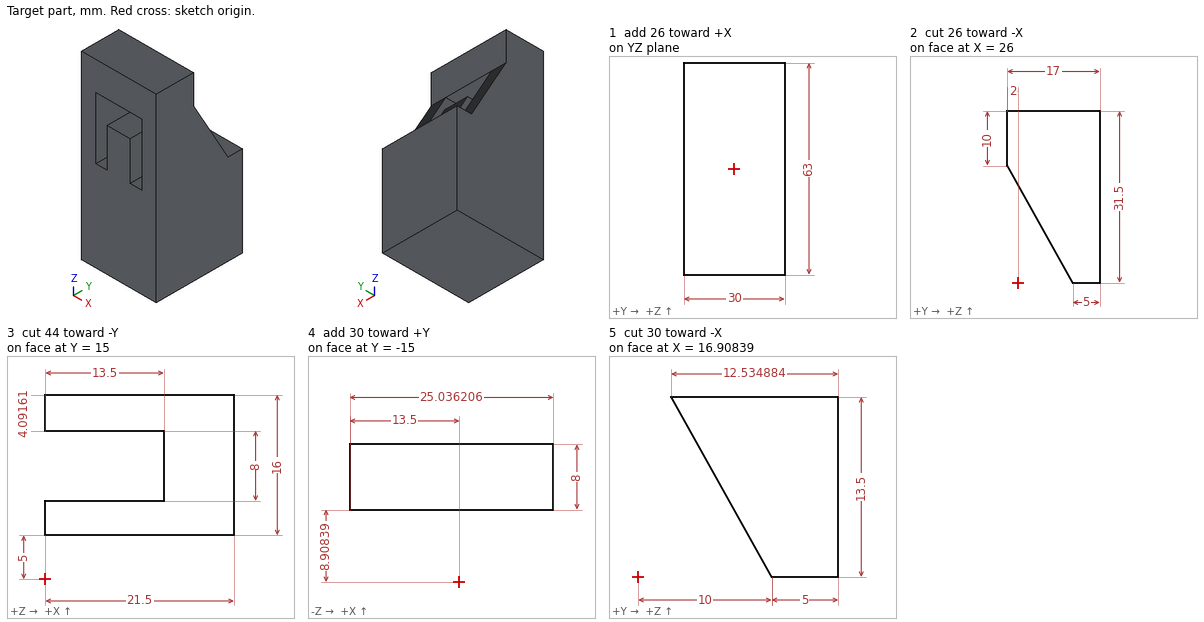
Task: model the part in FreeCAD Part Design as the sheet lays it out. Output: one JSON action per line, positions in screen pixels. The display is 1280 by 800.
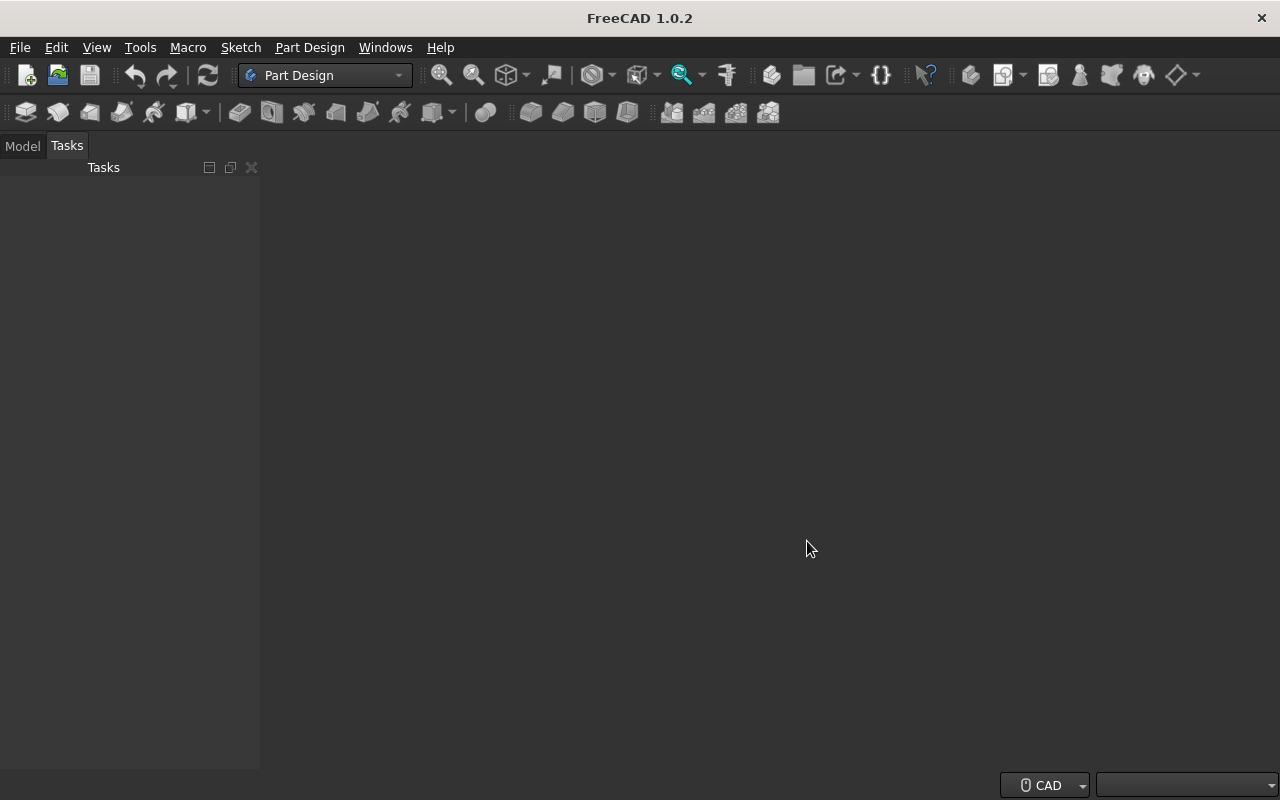
{"action": "key", "text": "ctrl+n"}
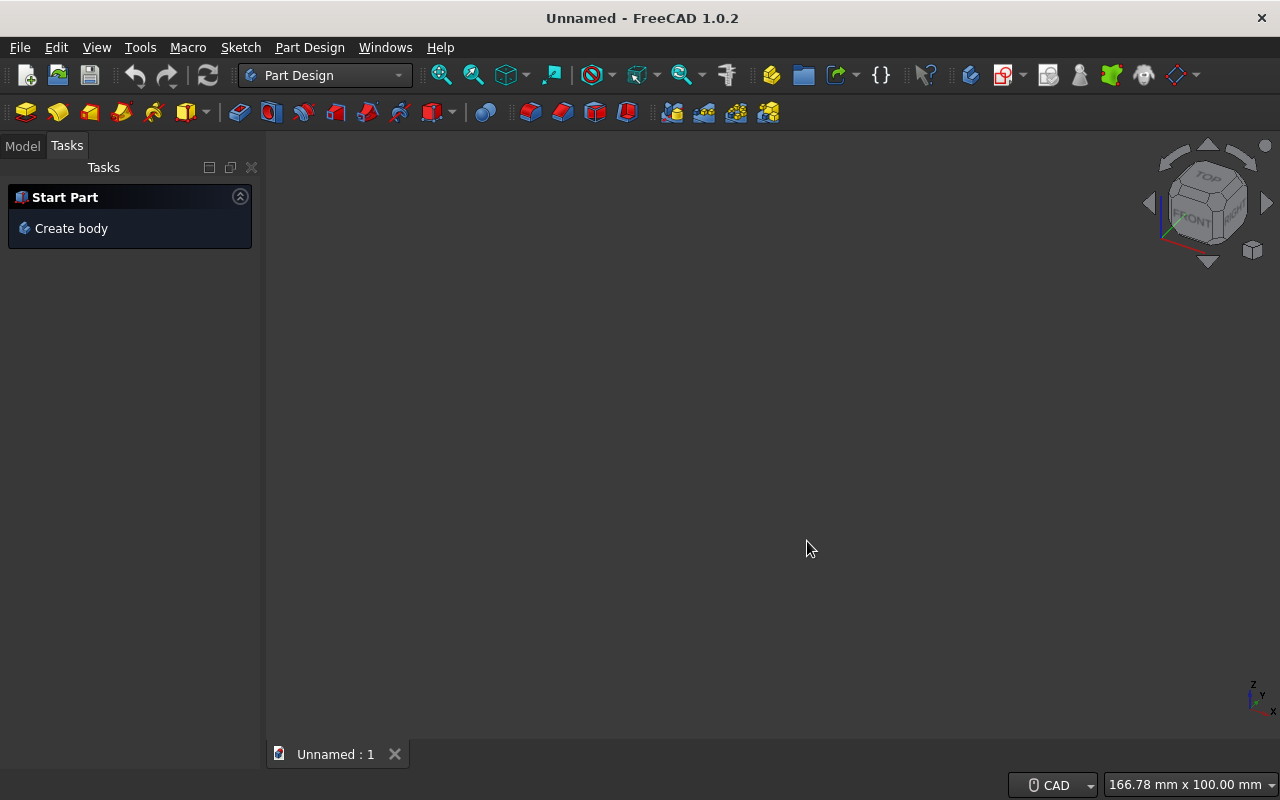
{"action": "left_click", "coordinate": [1004, 76]}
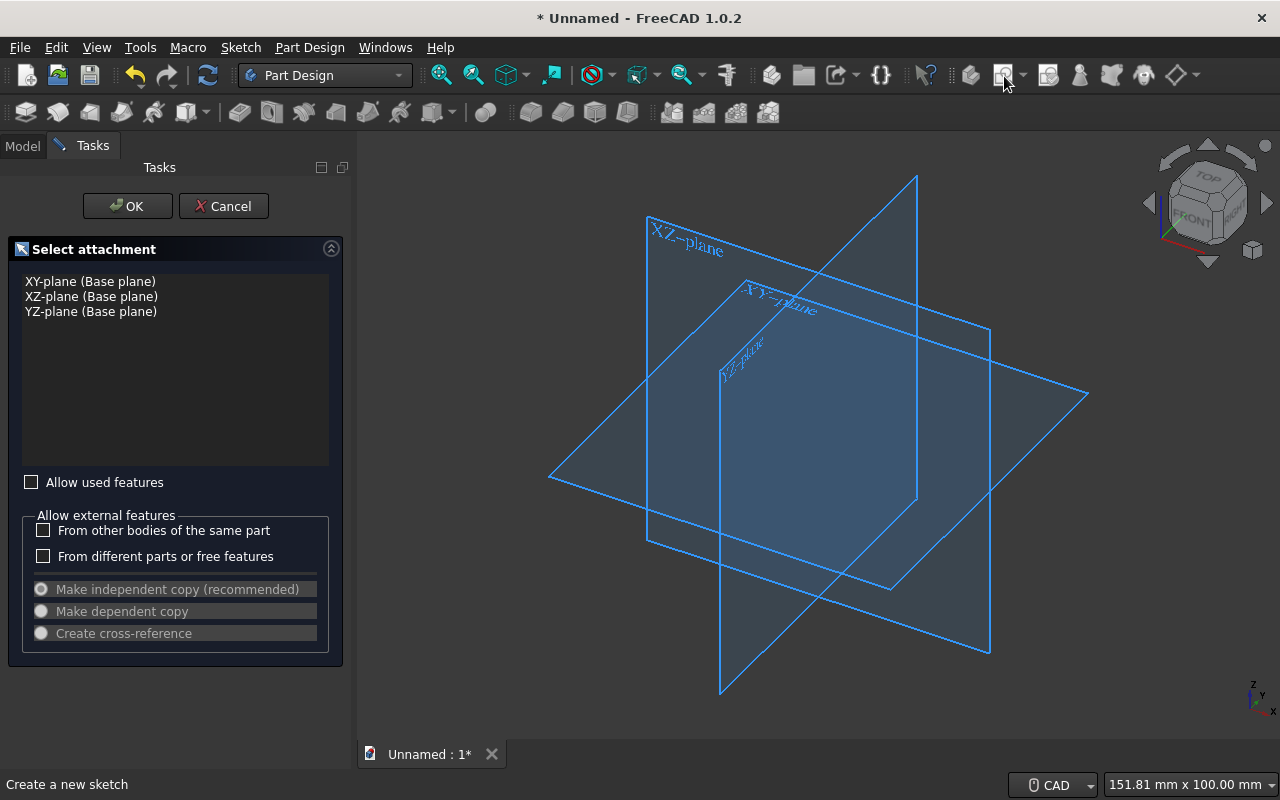
{"action": "left_click", "coordinate": [82, 312]}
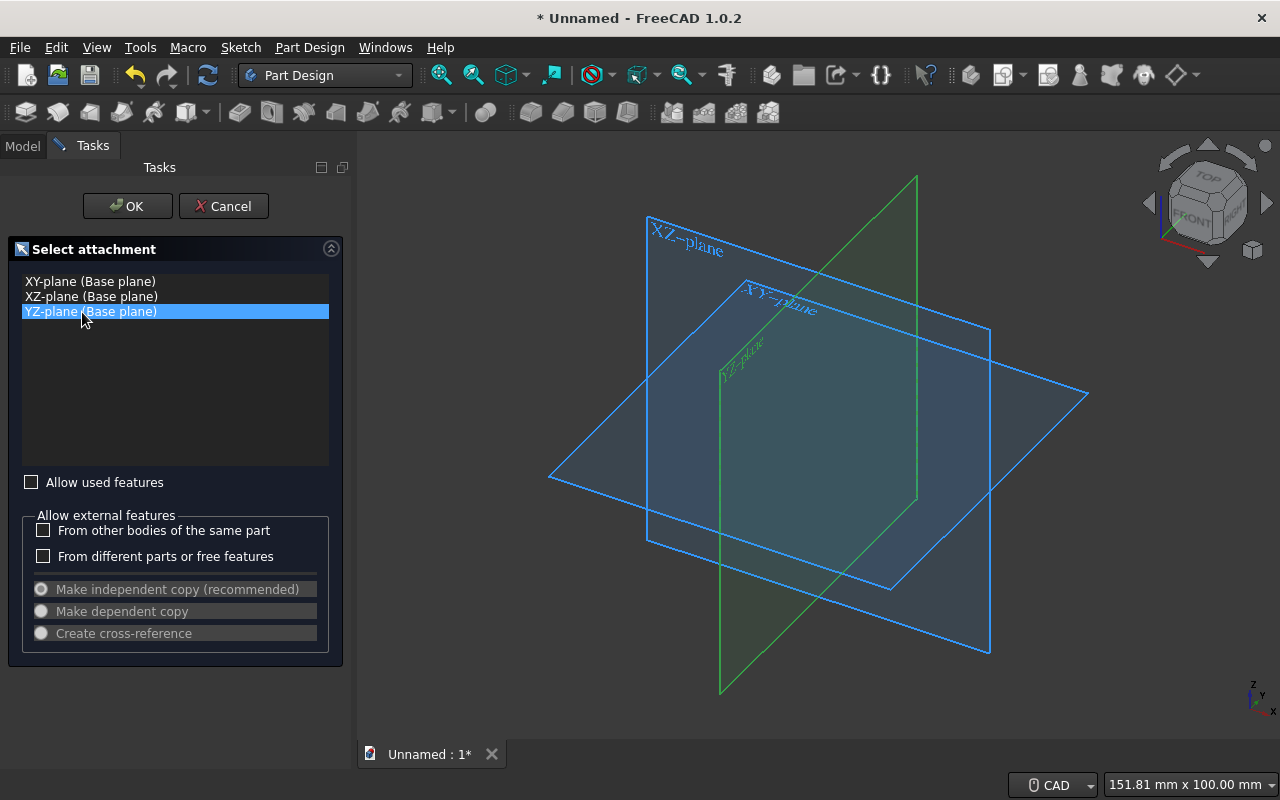
{"action": "left_click", "coordinate": [128, 206]}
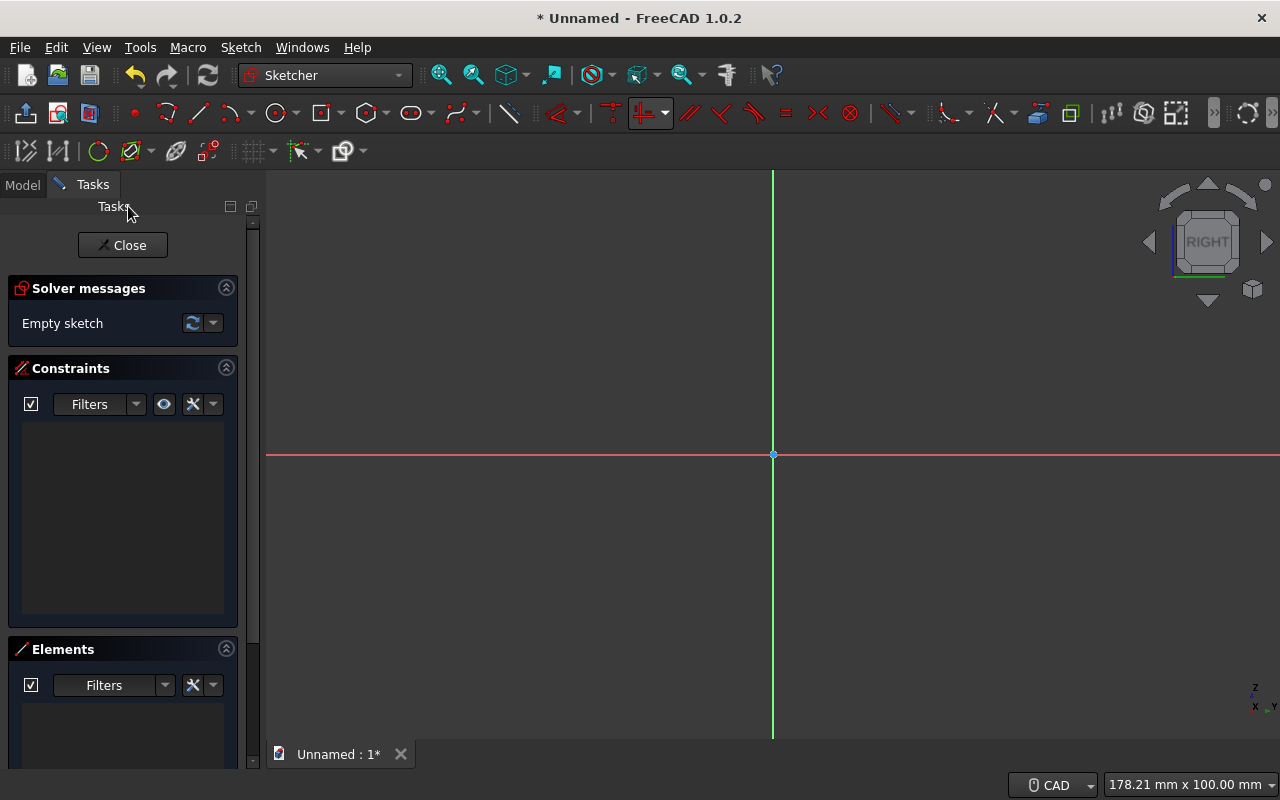
{"action": "key", "text": "g v"}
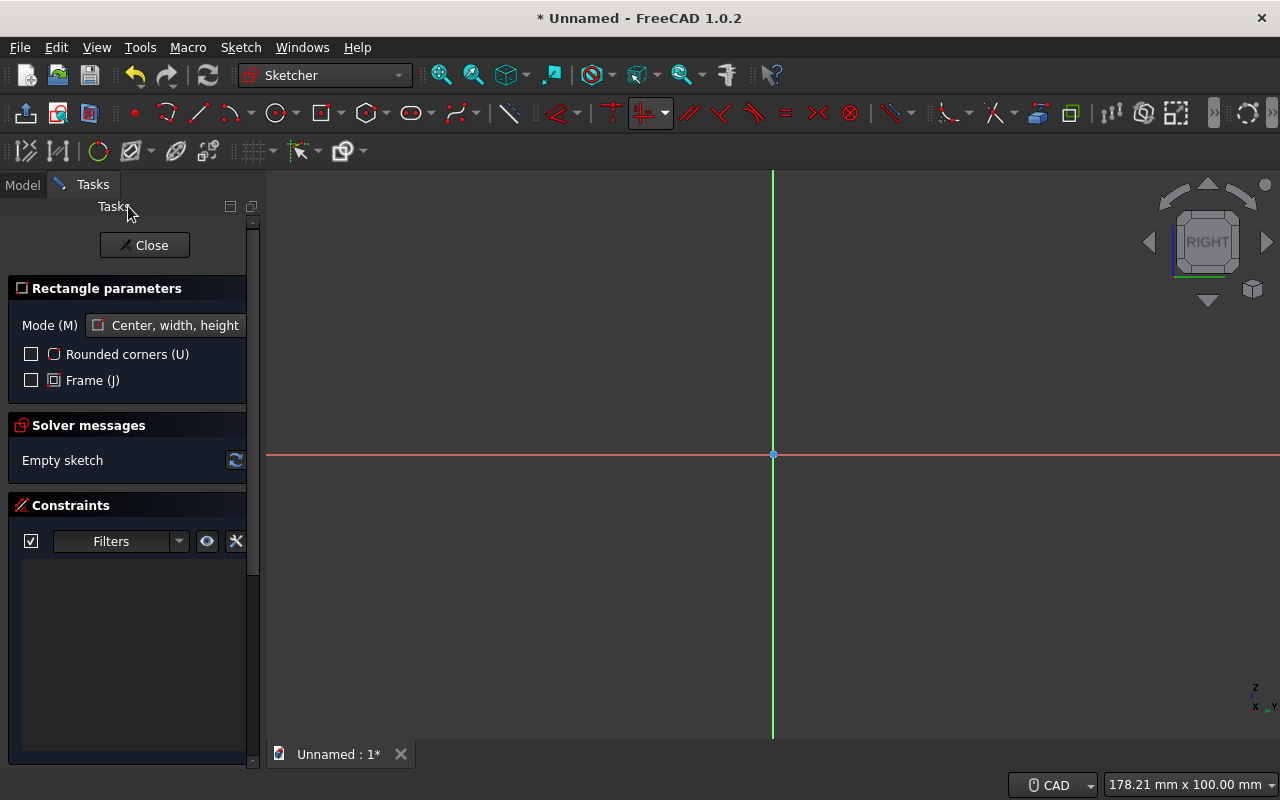
{"action": "left_click", "coordinate": [773, 454]}
{"action": "mouse_move", "coordinate": [858, 275]}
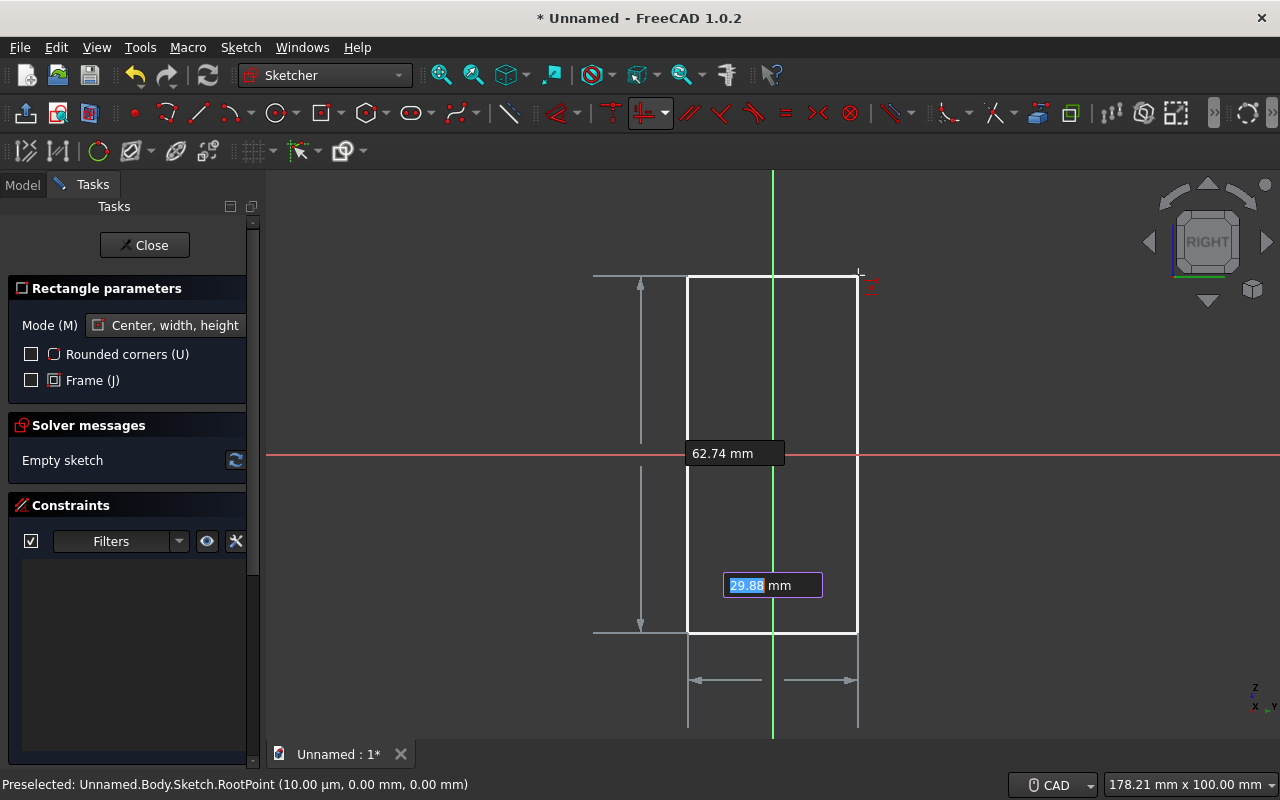
{"action": "type", "text": "30"}
{"action": "key", "text": "Tab"}
{"action": "type", "text": "63"}
{"action": "key", "text": "Return"}
{"action": "key", "text": "Escape"}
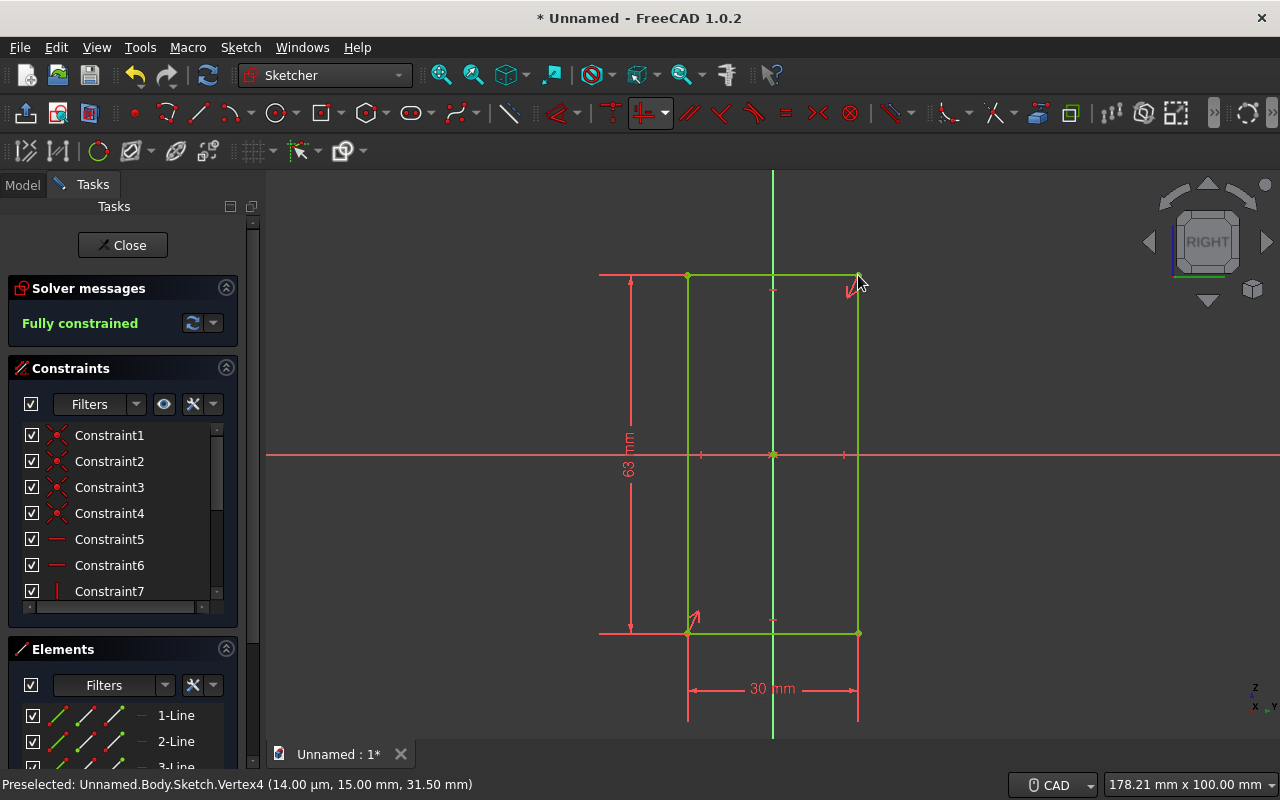
{"action": "left_click", "coordinate": [123, 245]}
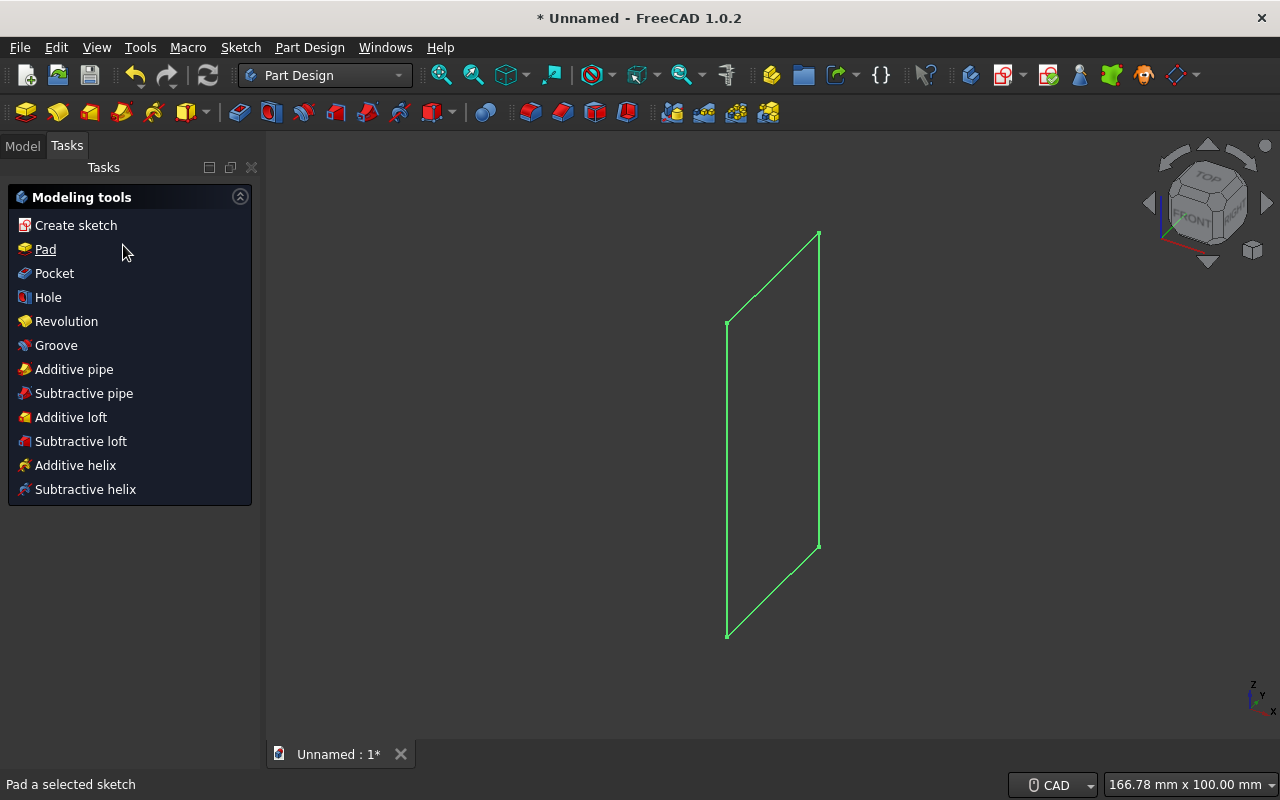
{"action": "left_click", "coordinate": [26, 112]}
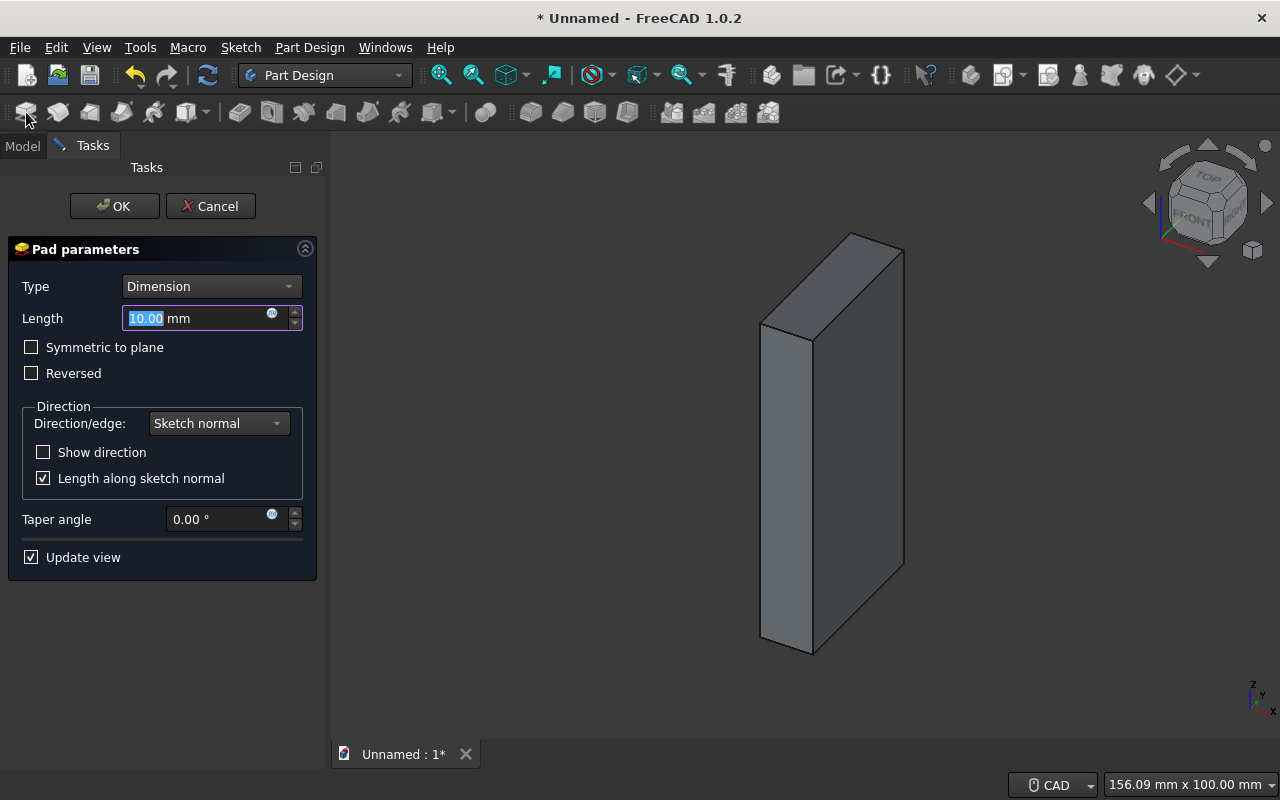
{"action": "type", "text": "26"}
{"action": "key", "text": "Tab"}